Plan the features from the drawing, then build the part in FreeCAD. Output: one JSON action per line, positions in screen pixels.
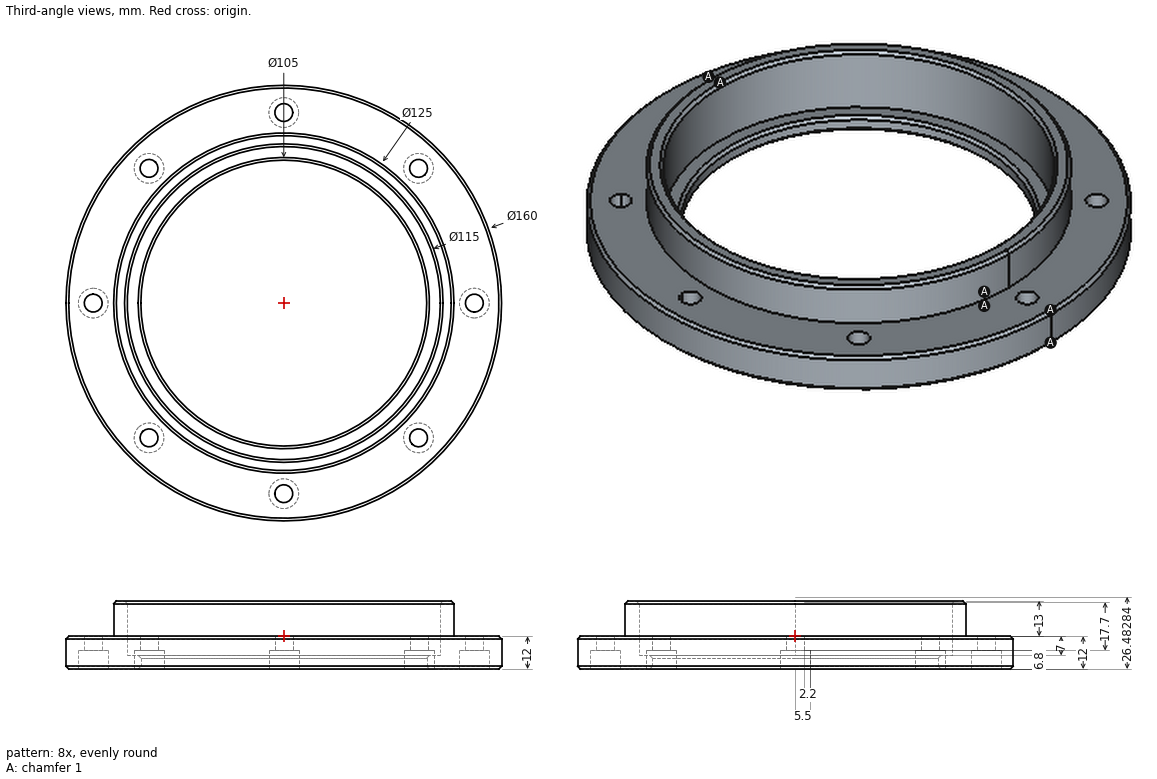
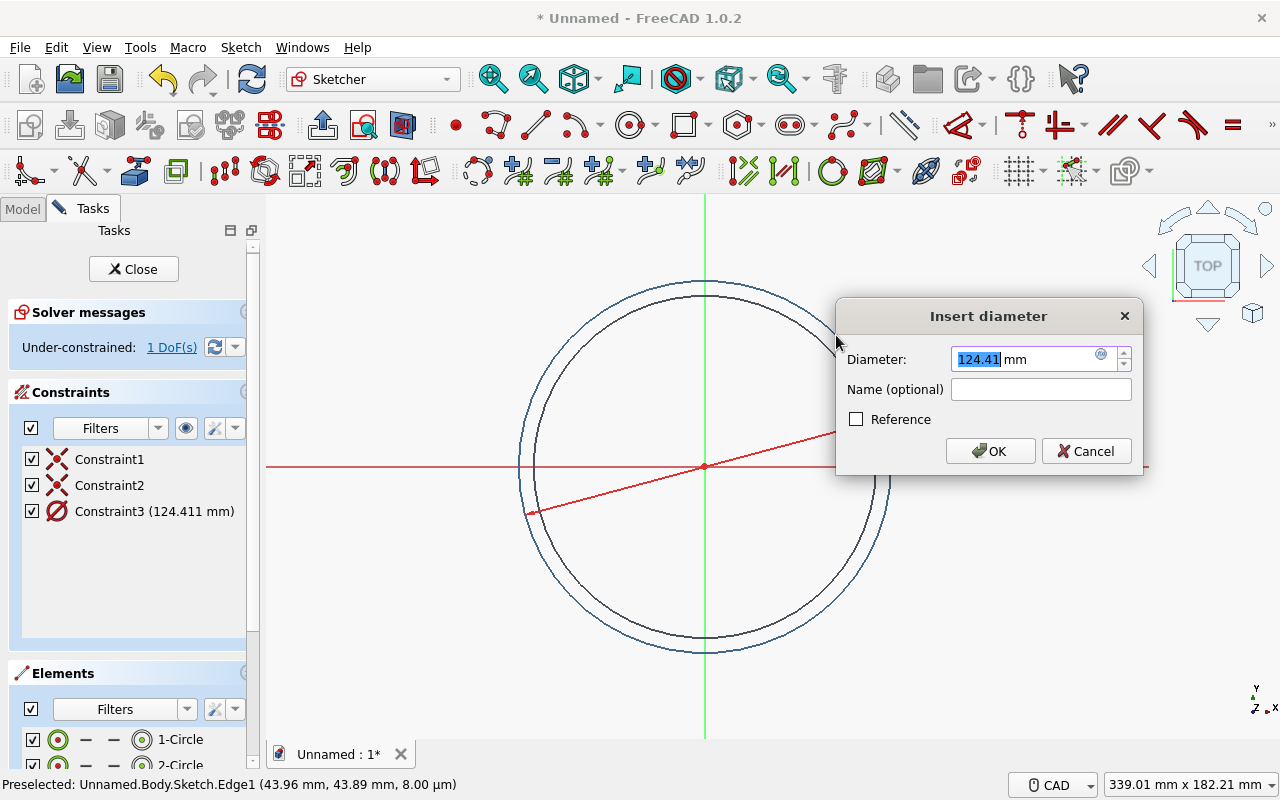
{"action": "type", "text": "125"}
{"action": "key", "text": "Return"}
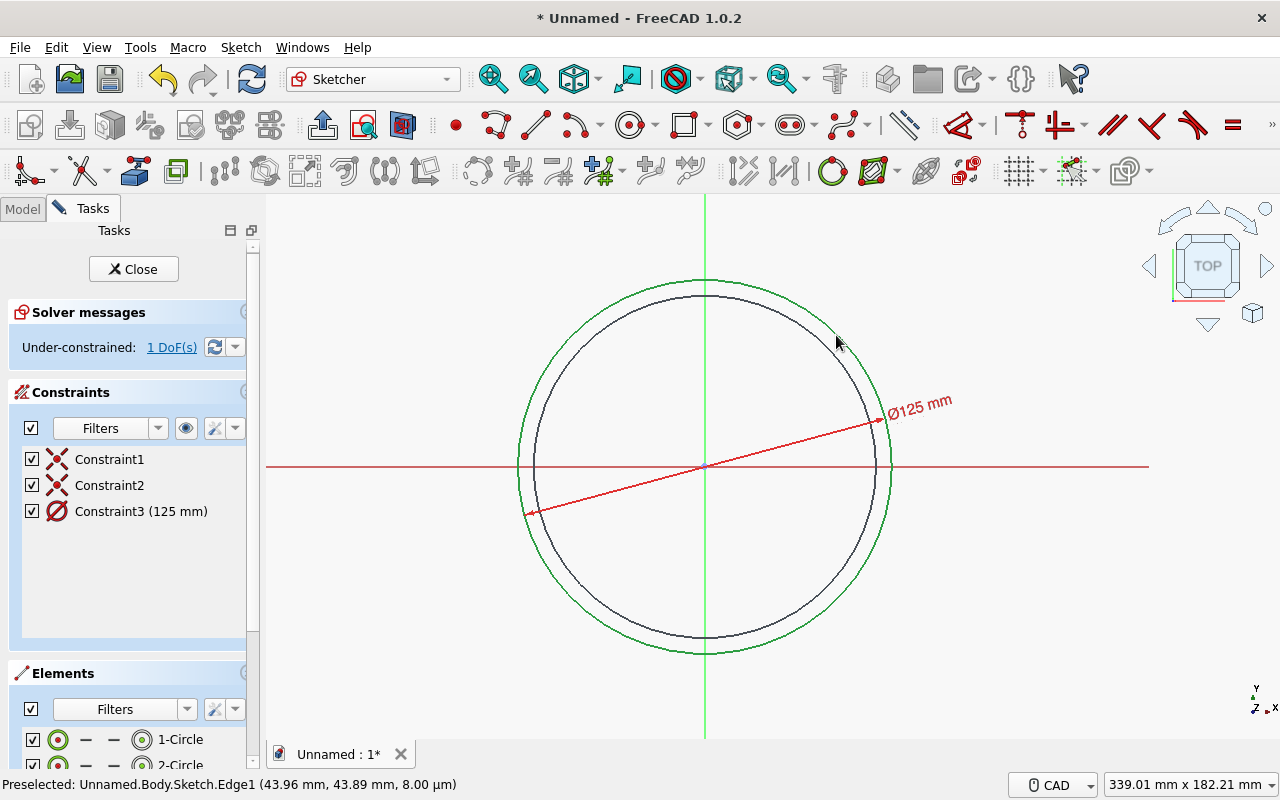
{"action": "left_click", "coordinate": [826, 346]}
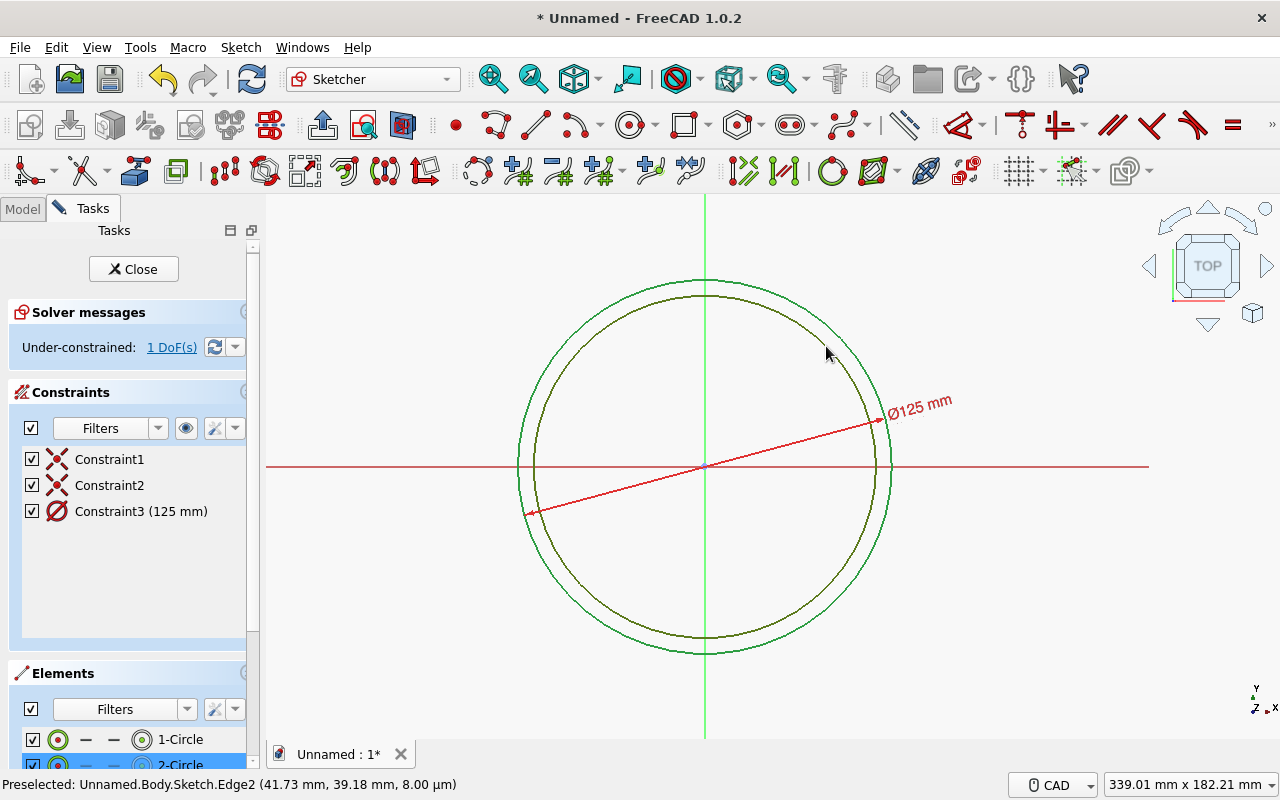
{"action": "key", "text": "k o"}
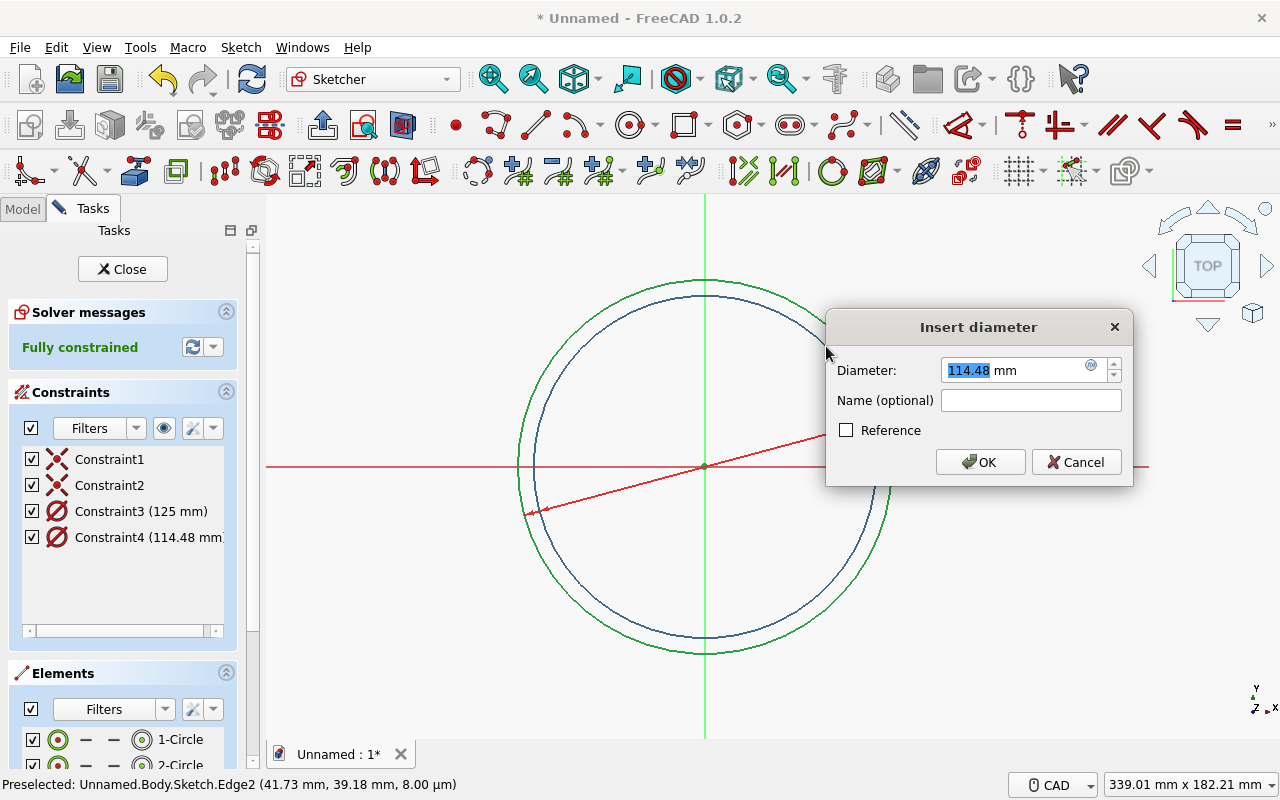
{"action": "type", "text": "115"}
{"action": "key", "text": "Return"}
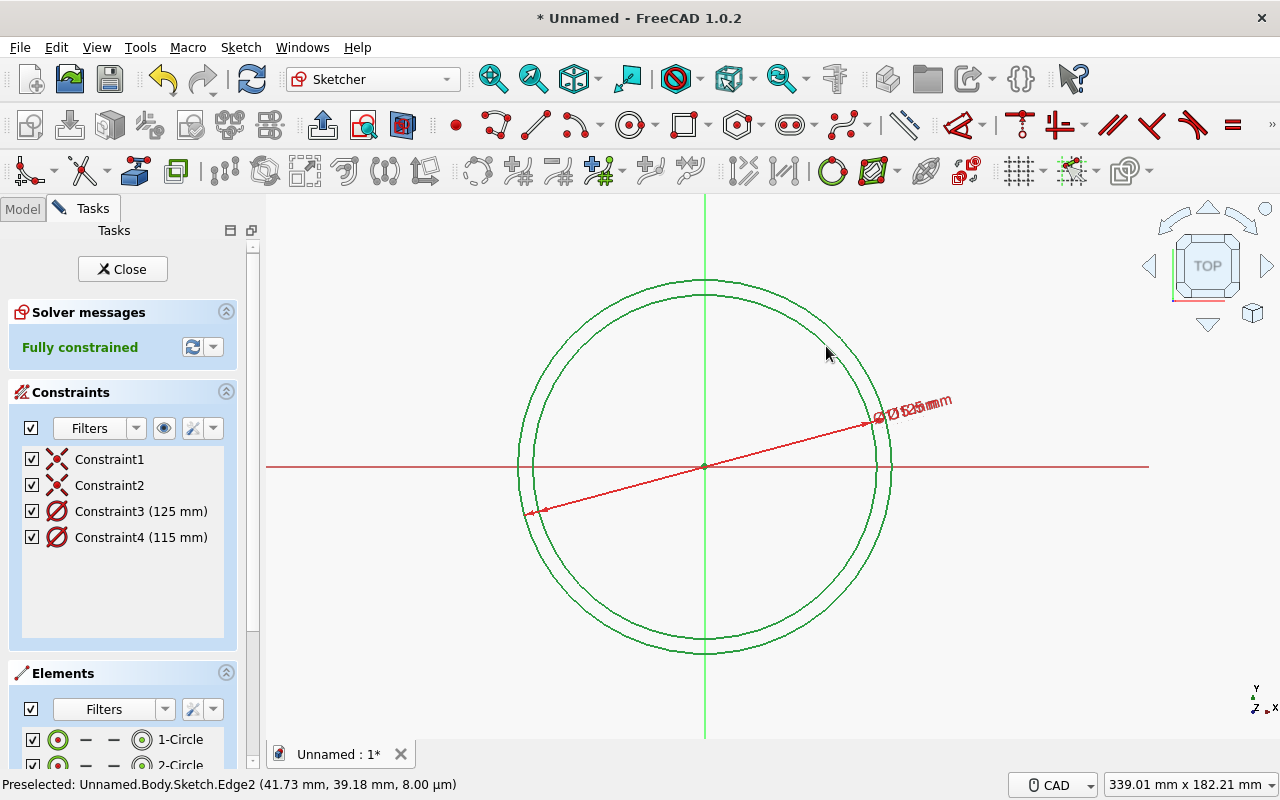
{"action": "left_click", "coordinate": [123, 269]}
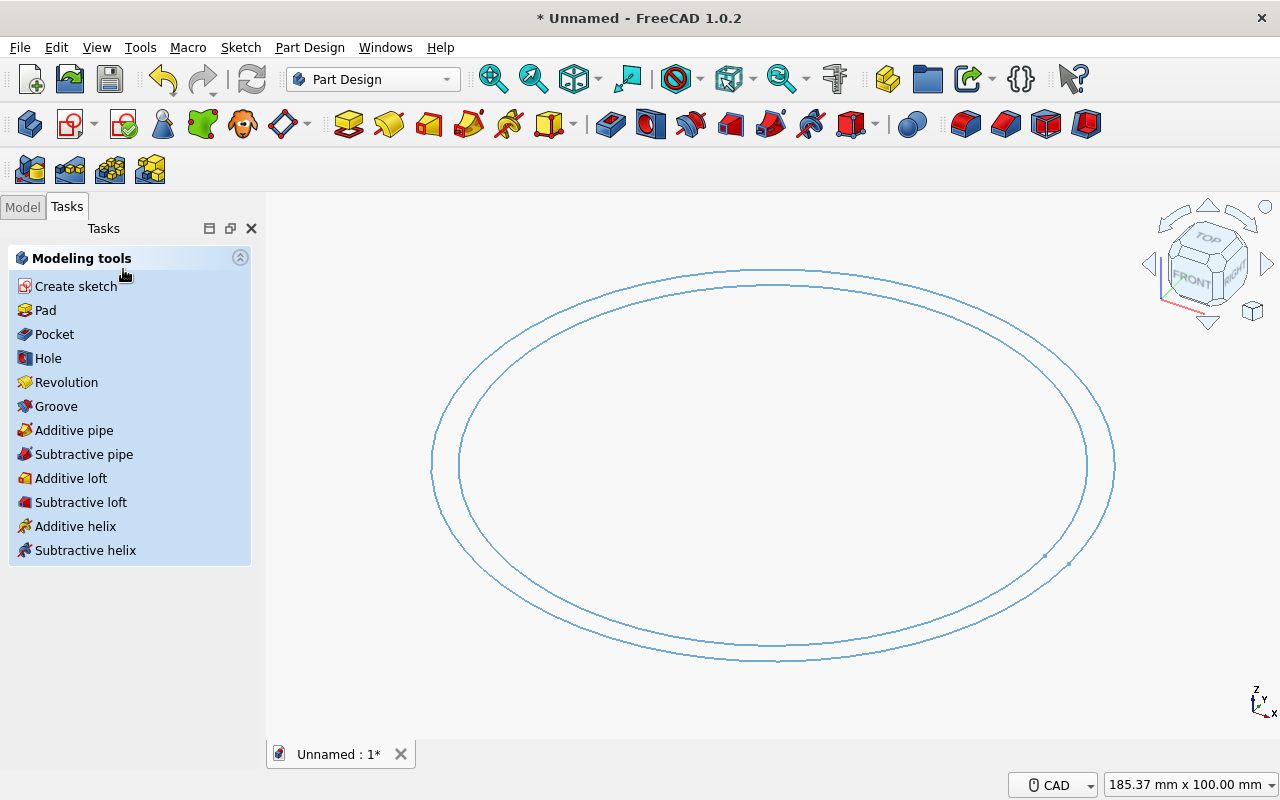
{"action": "left_click", "coordinate": [350, 124]}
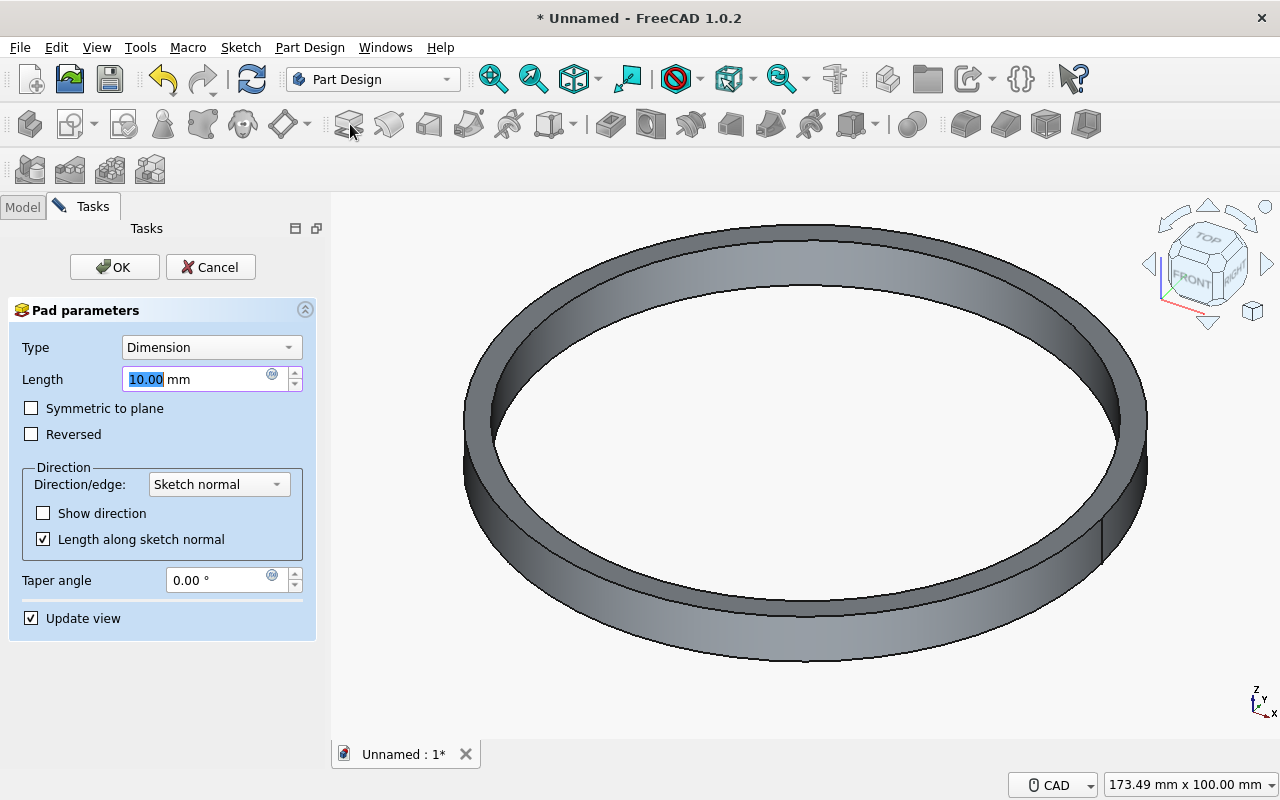
{"action": "type", "text": "13"}
{"action": "key", "text": "Tab"}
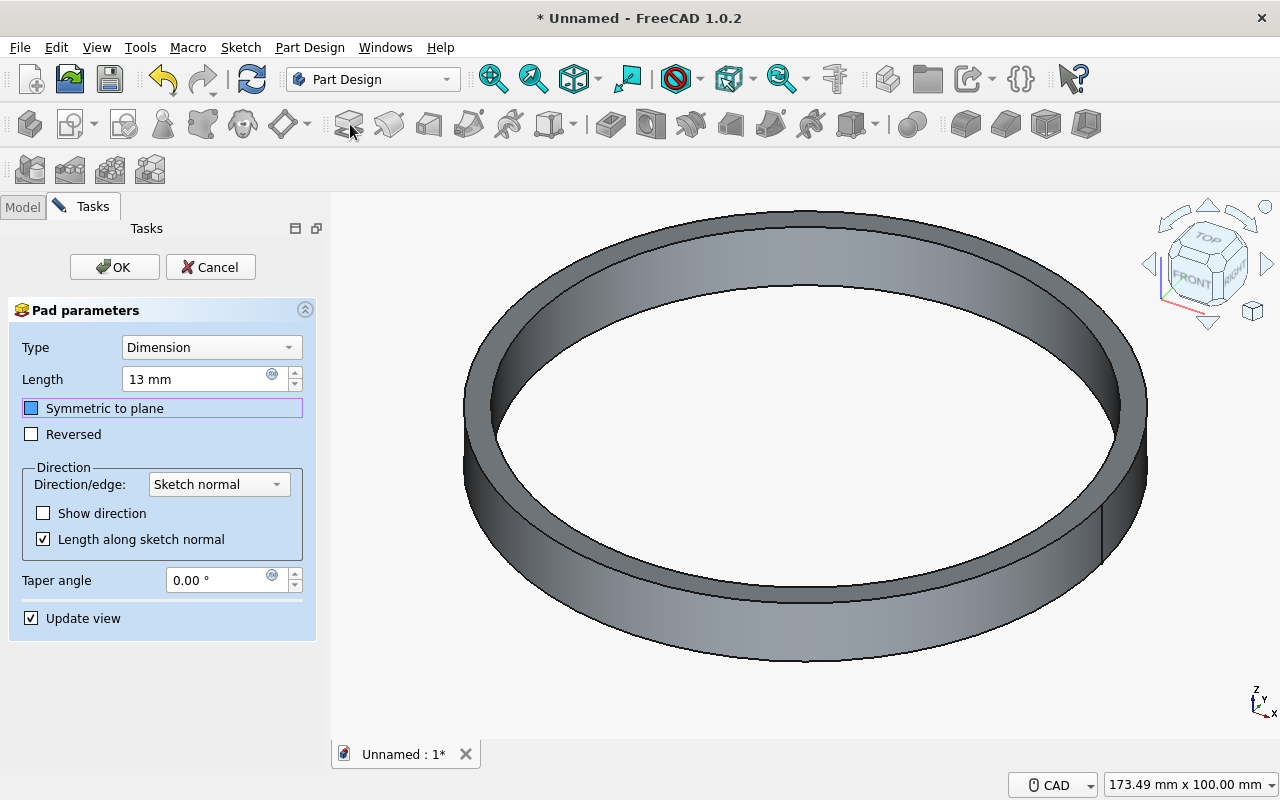
{"action": "left_click", "coordinate": [115, 267]}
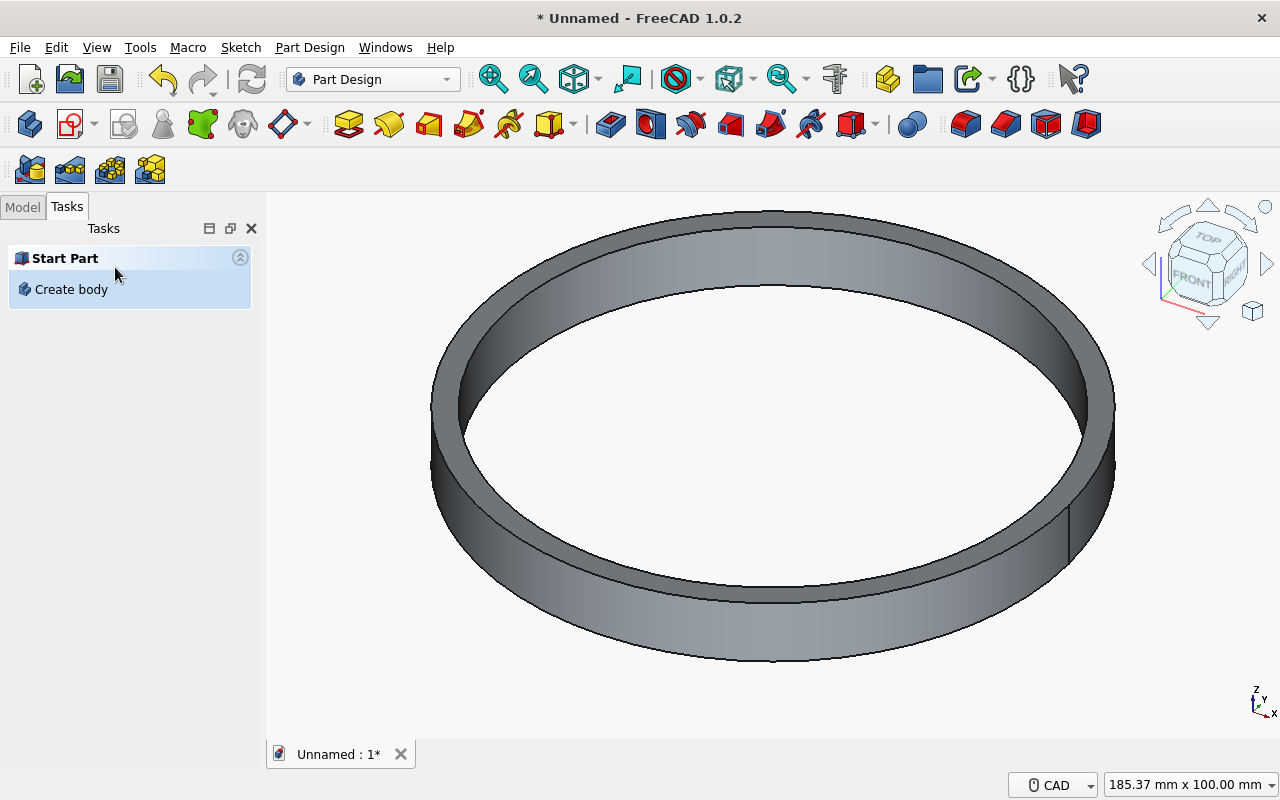
{"action": "key", "text": "v f"}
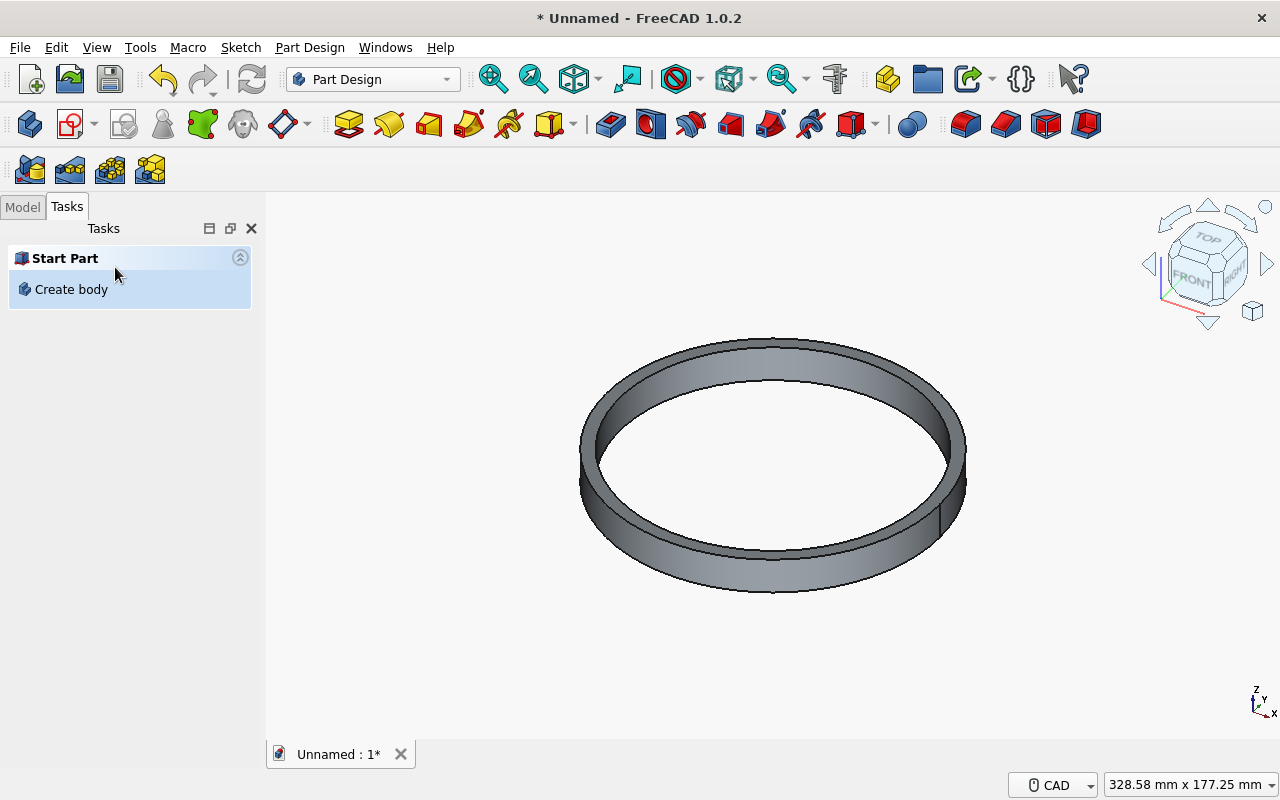
{"action": "key", "text": "5"}